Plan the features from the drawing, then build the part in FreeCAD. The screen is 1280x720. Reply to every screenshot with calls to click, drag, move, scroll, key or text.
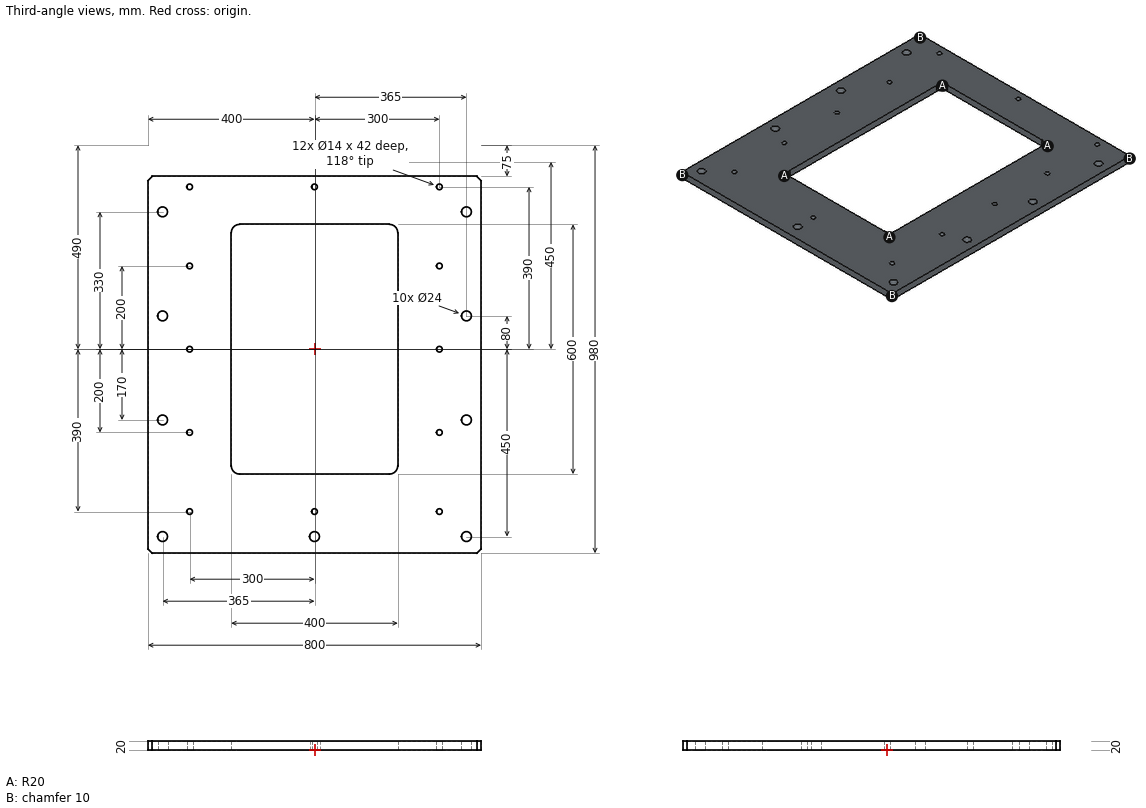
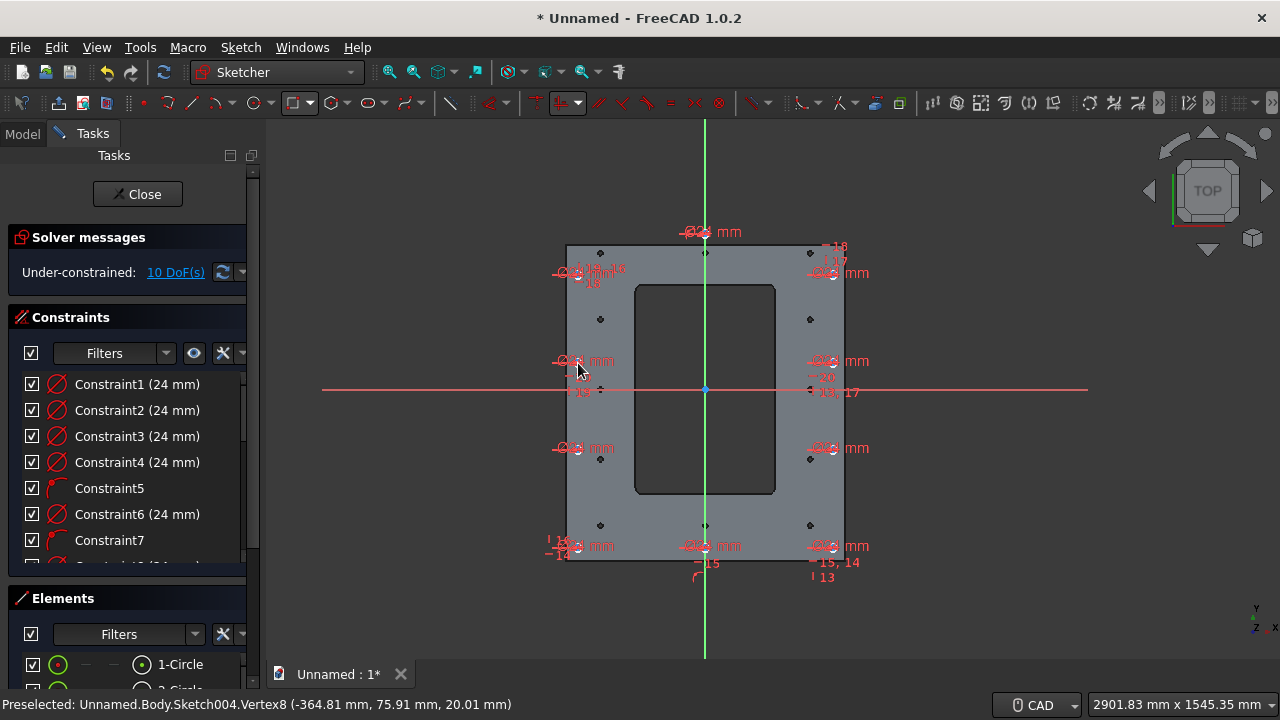
click(578, 363)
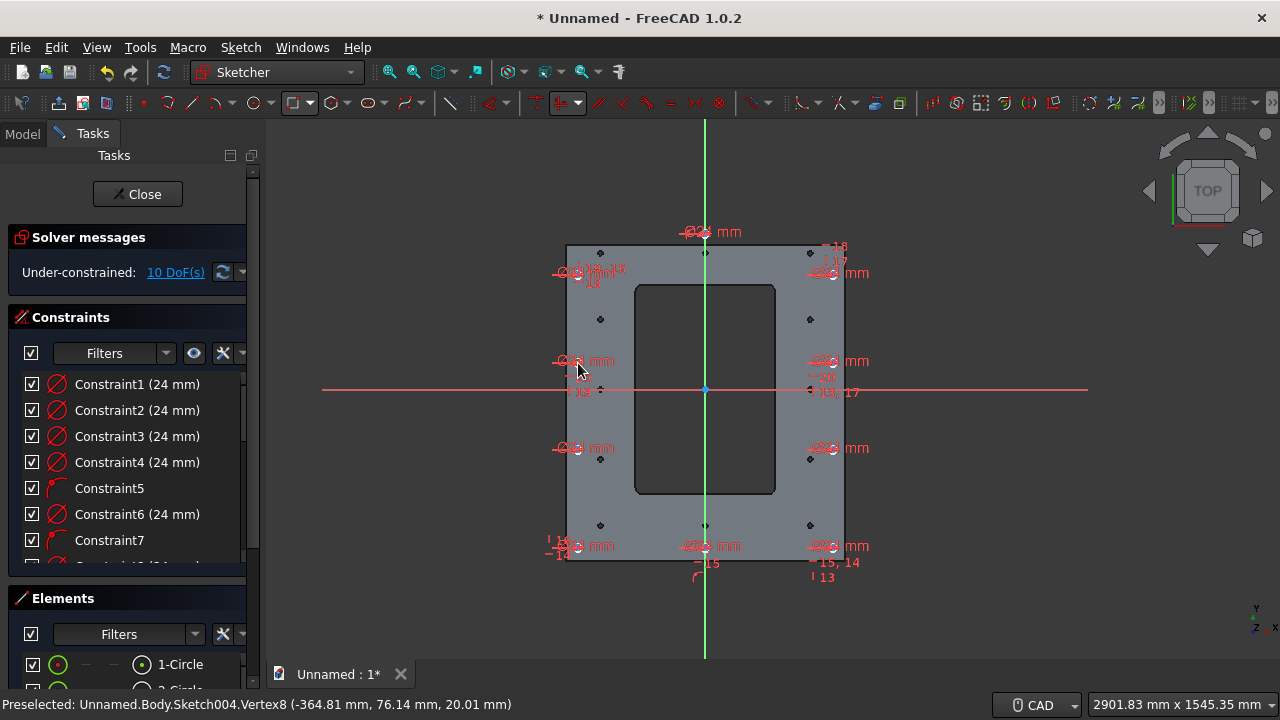
click(578, 450)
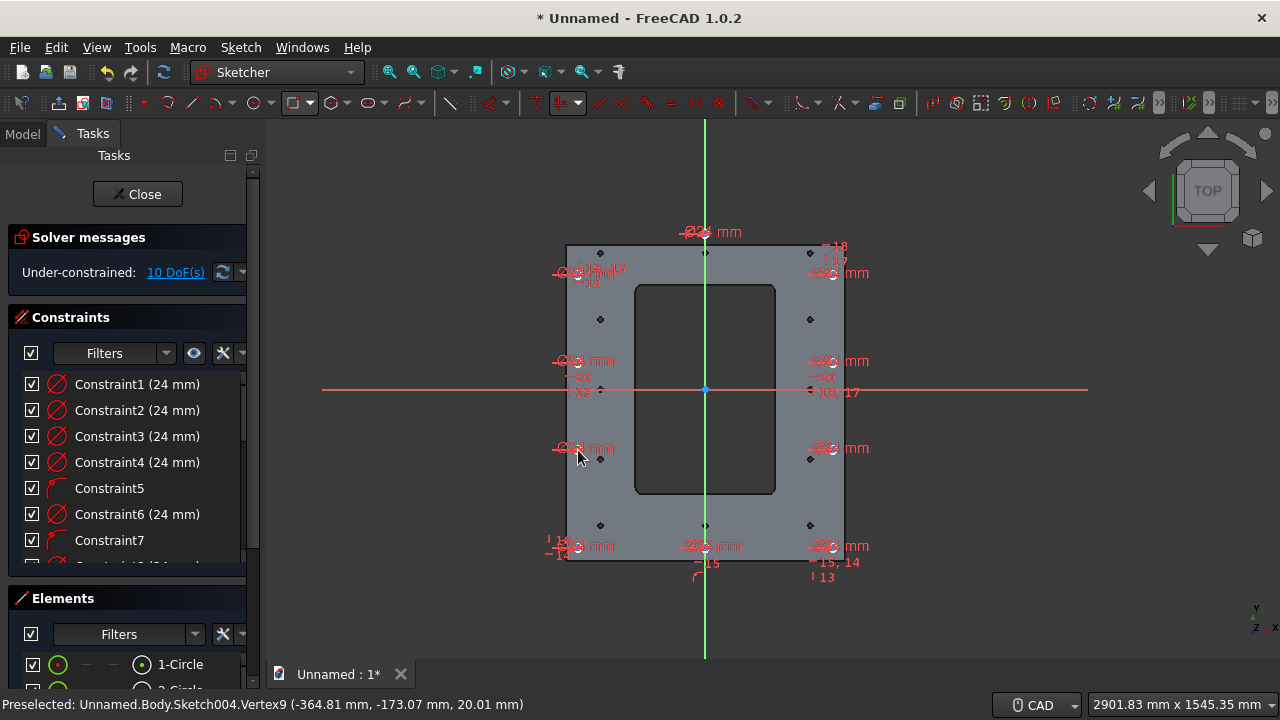
click(580, 104)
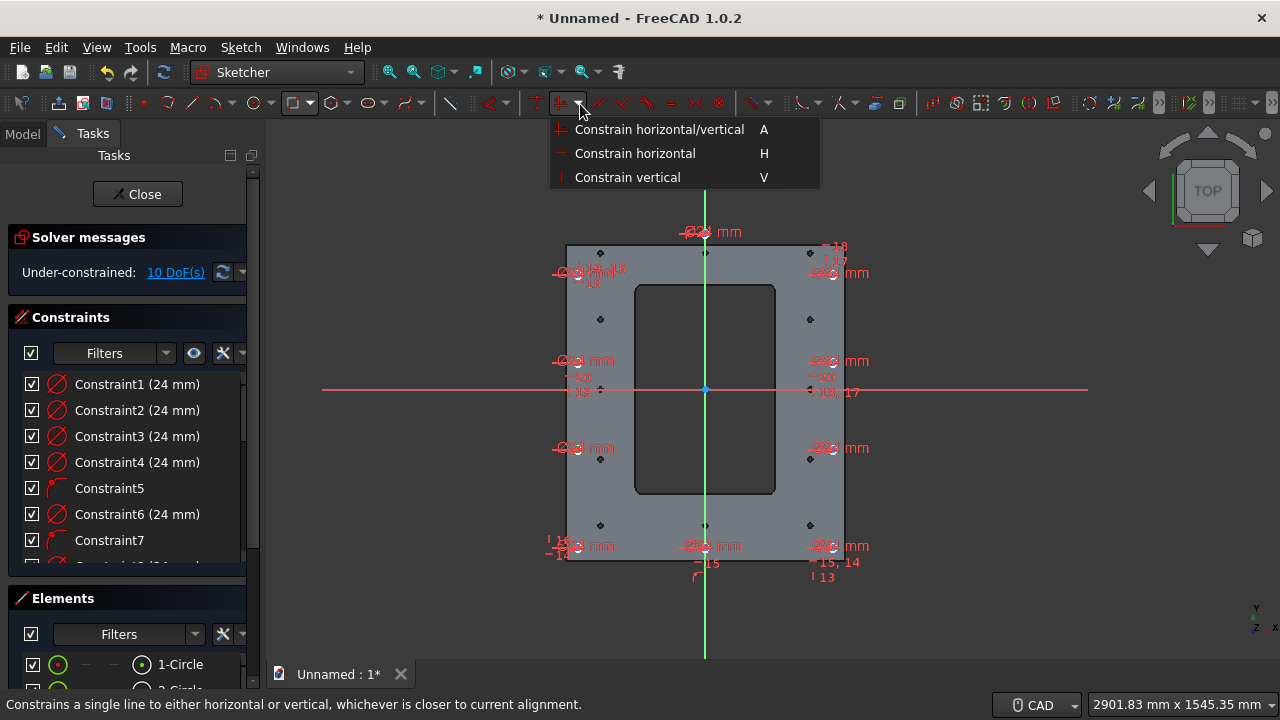
click(685, 177)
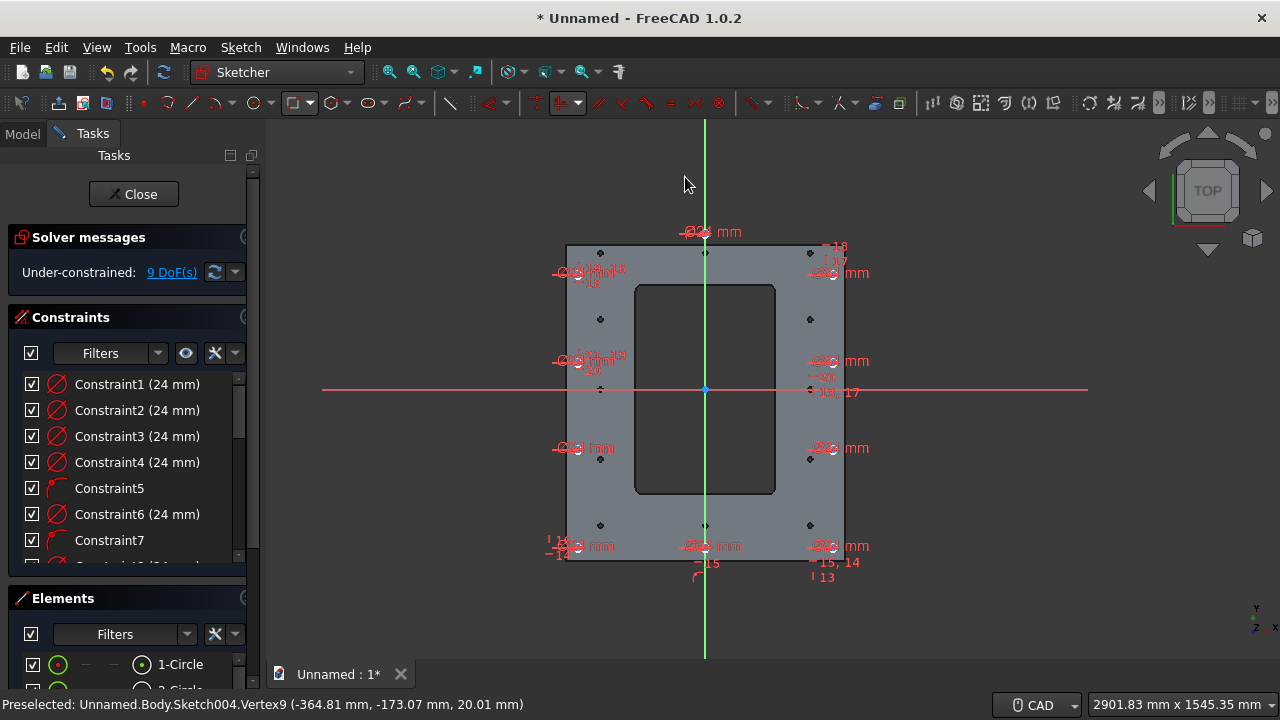
click(833, 363)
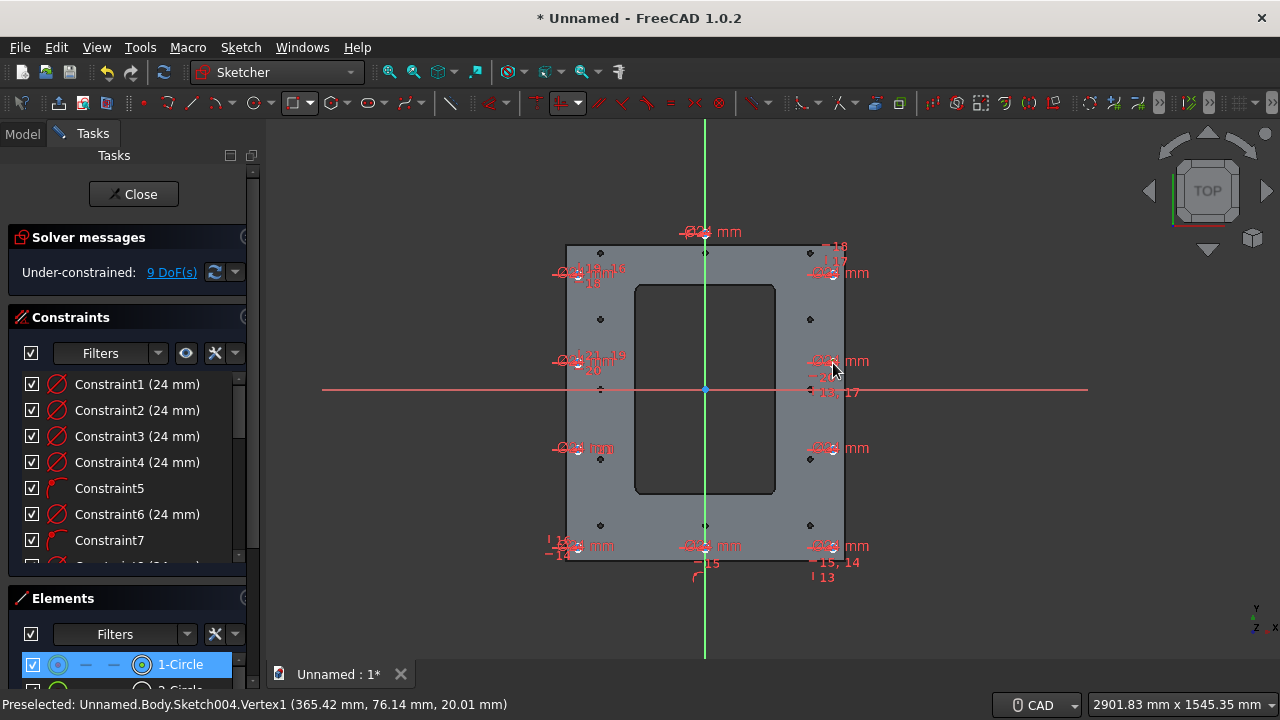
click(833, 450)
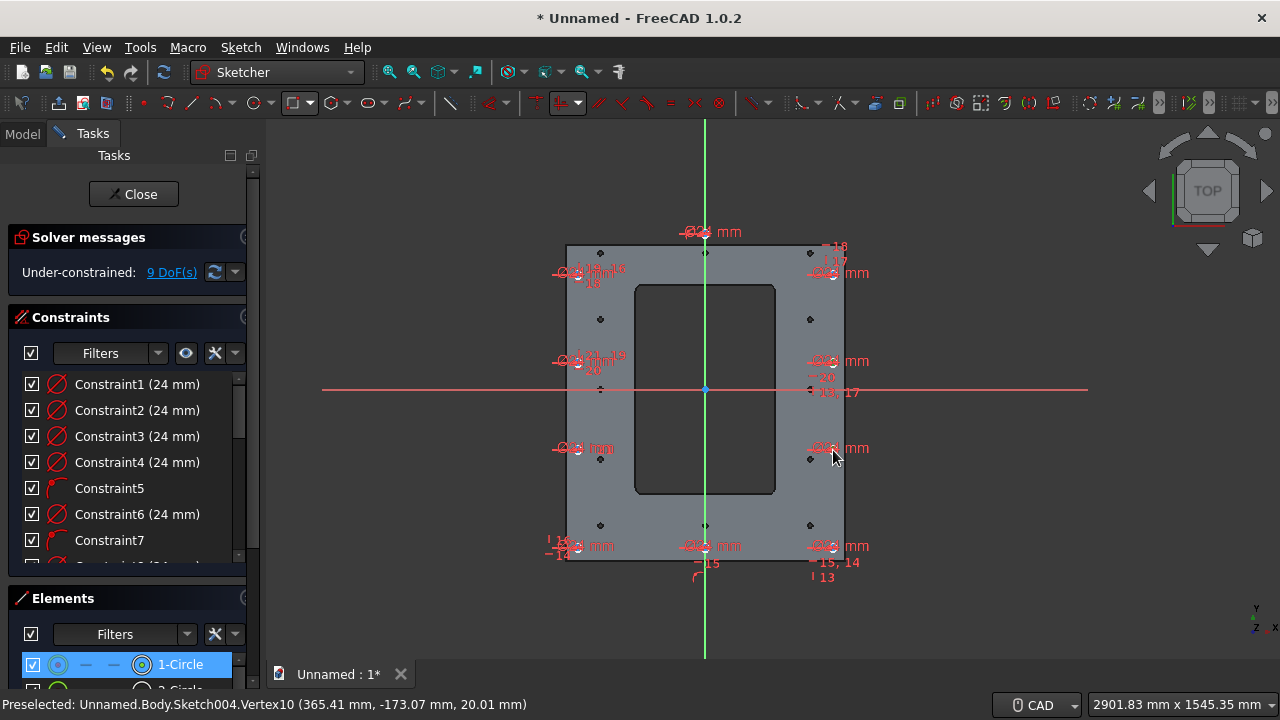
key(v)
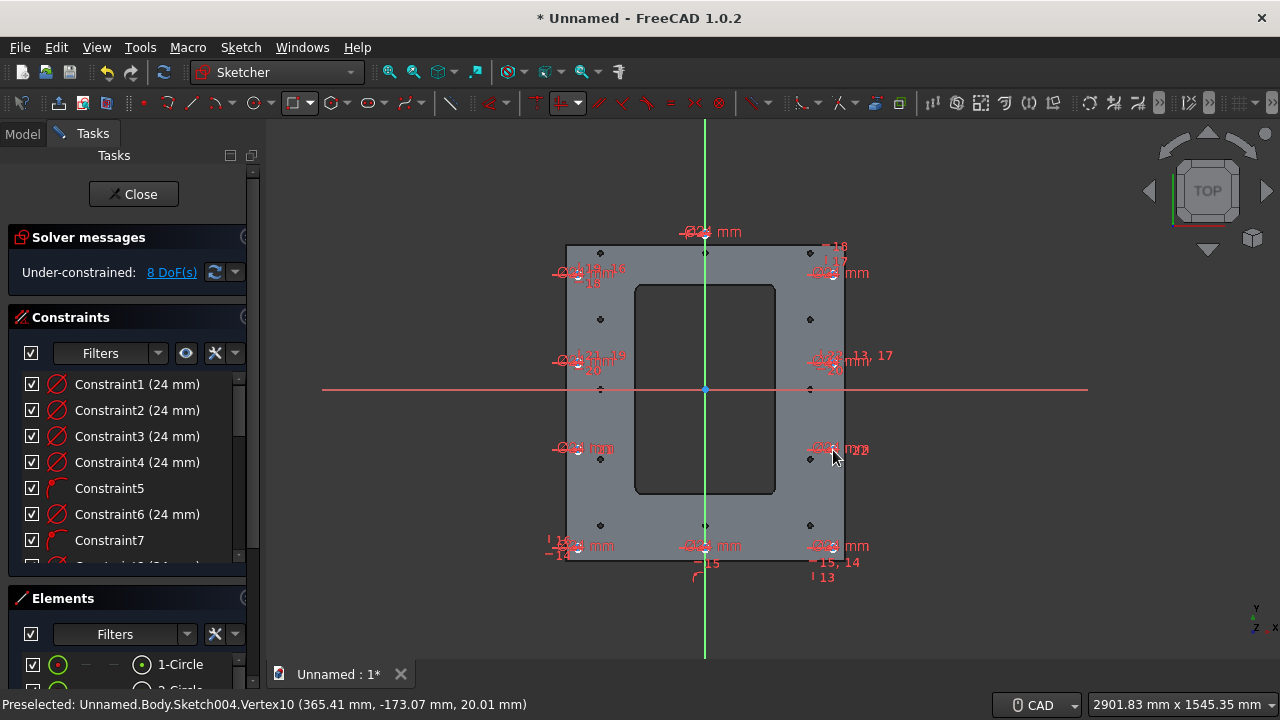
click(578, 450)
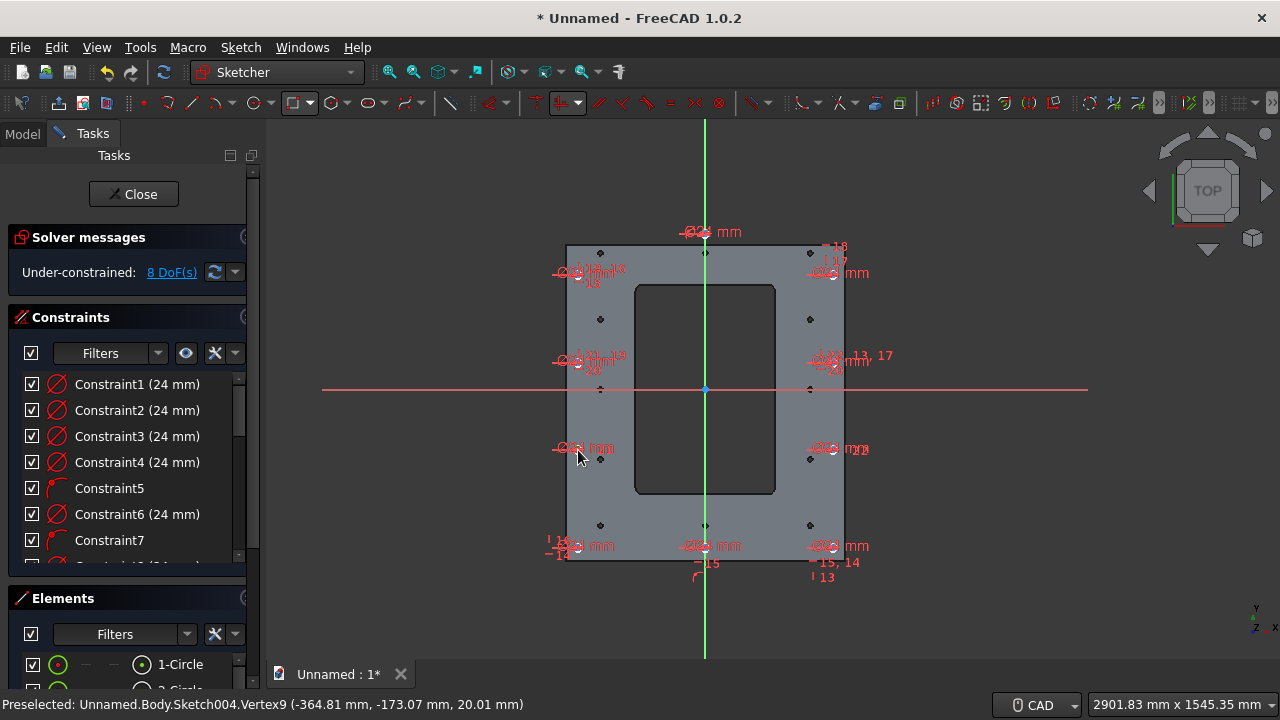
click(833, 450)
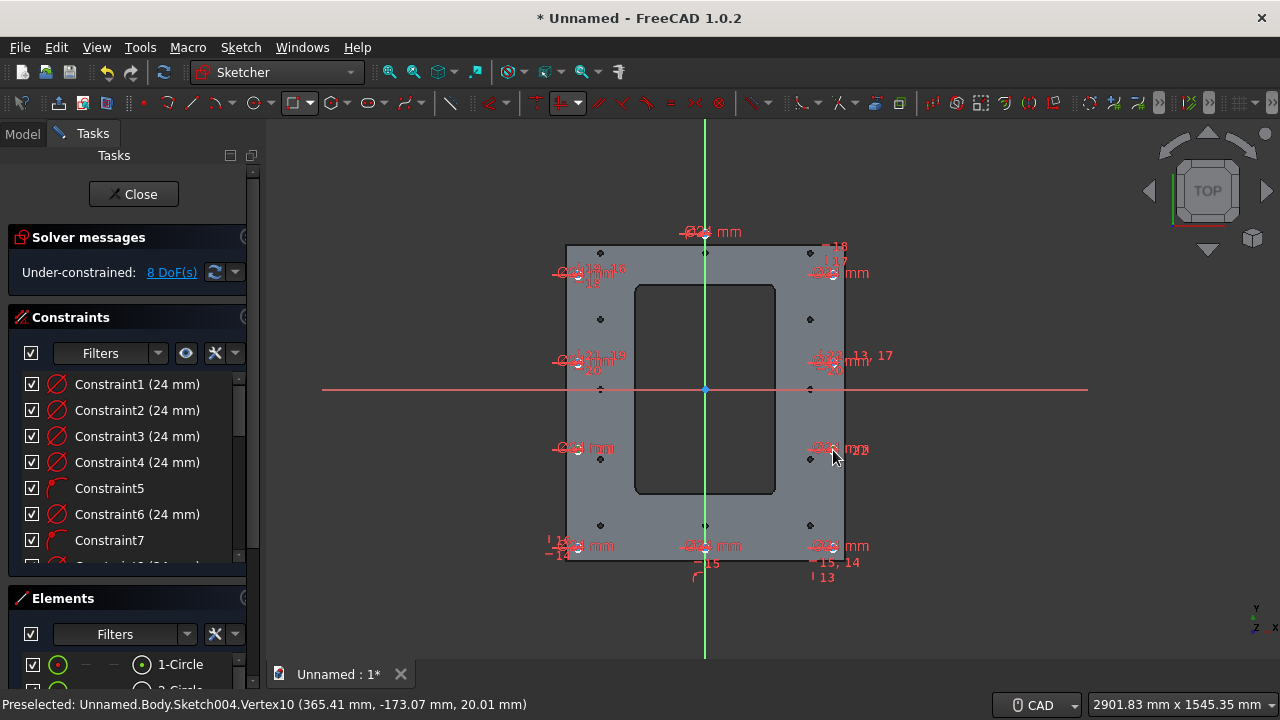
click(580, 104)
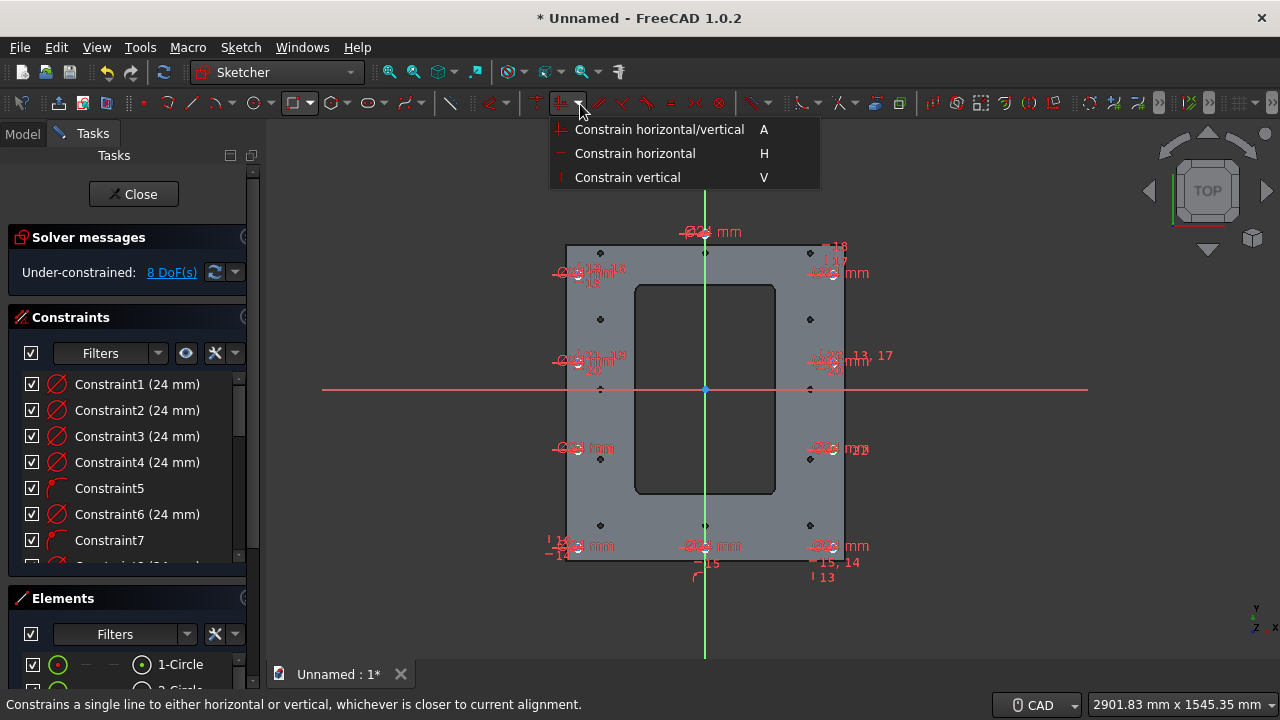
click(685, 153)